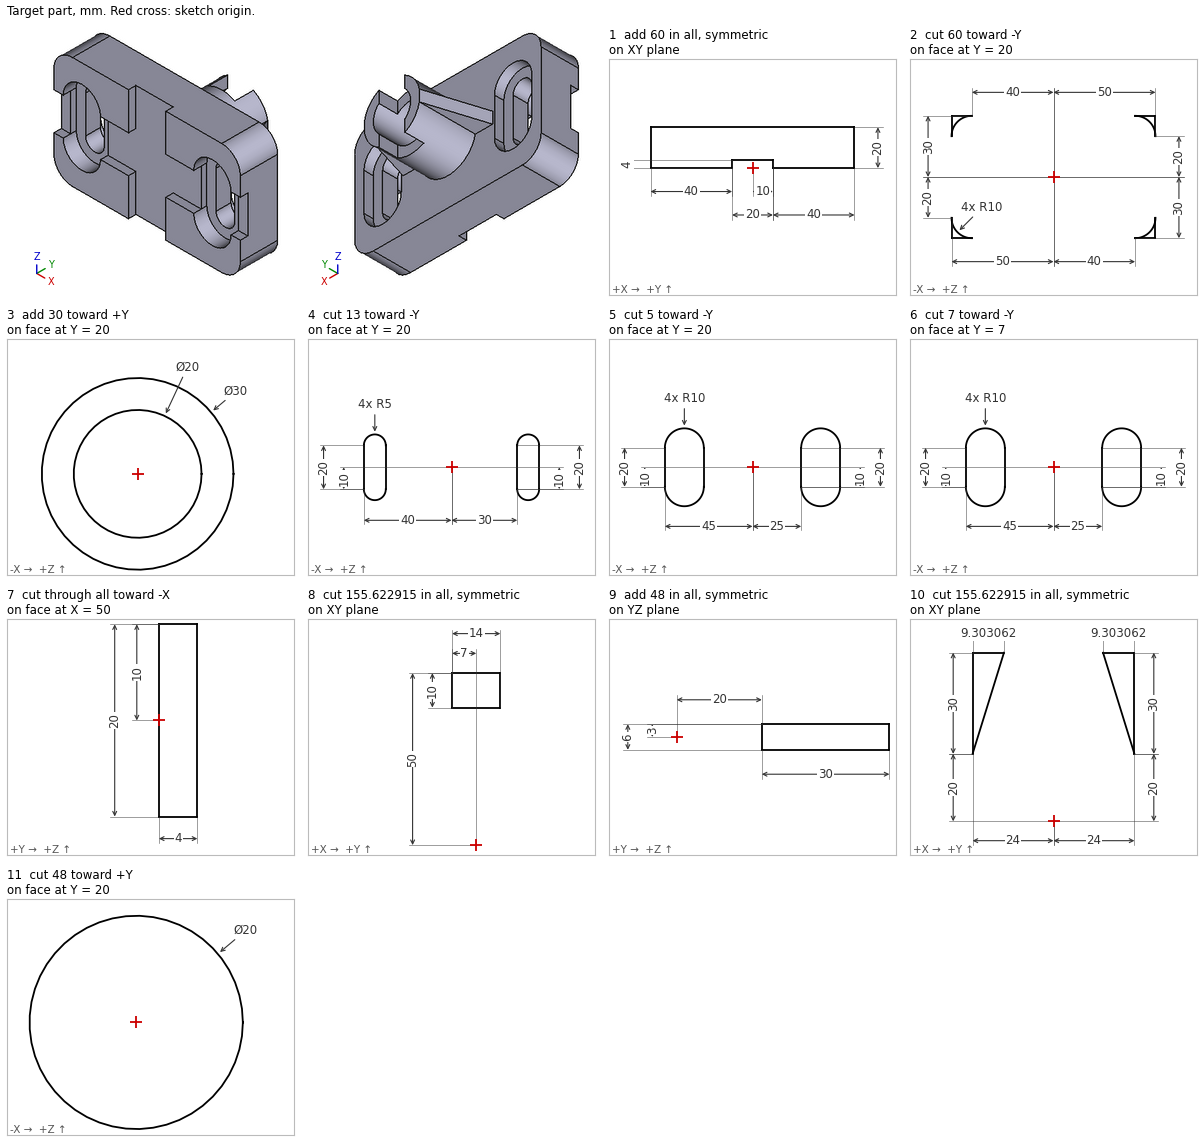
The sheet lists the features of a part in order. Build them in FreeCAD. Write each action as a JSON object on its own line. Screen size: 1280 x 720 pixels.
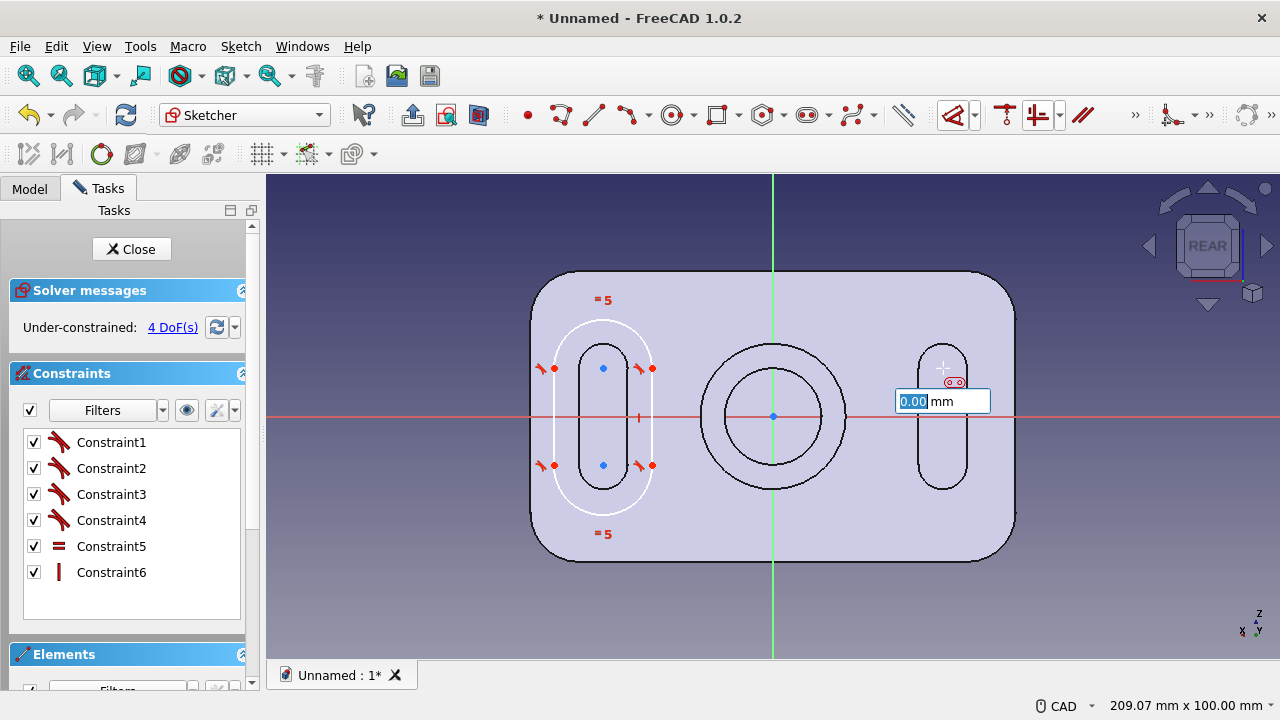
{"action": "left_click", "coordinate": [894, 402]}
{"action": "key", "text": "Escape"}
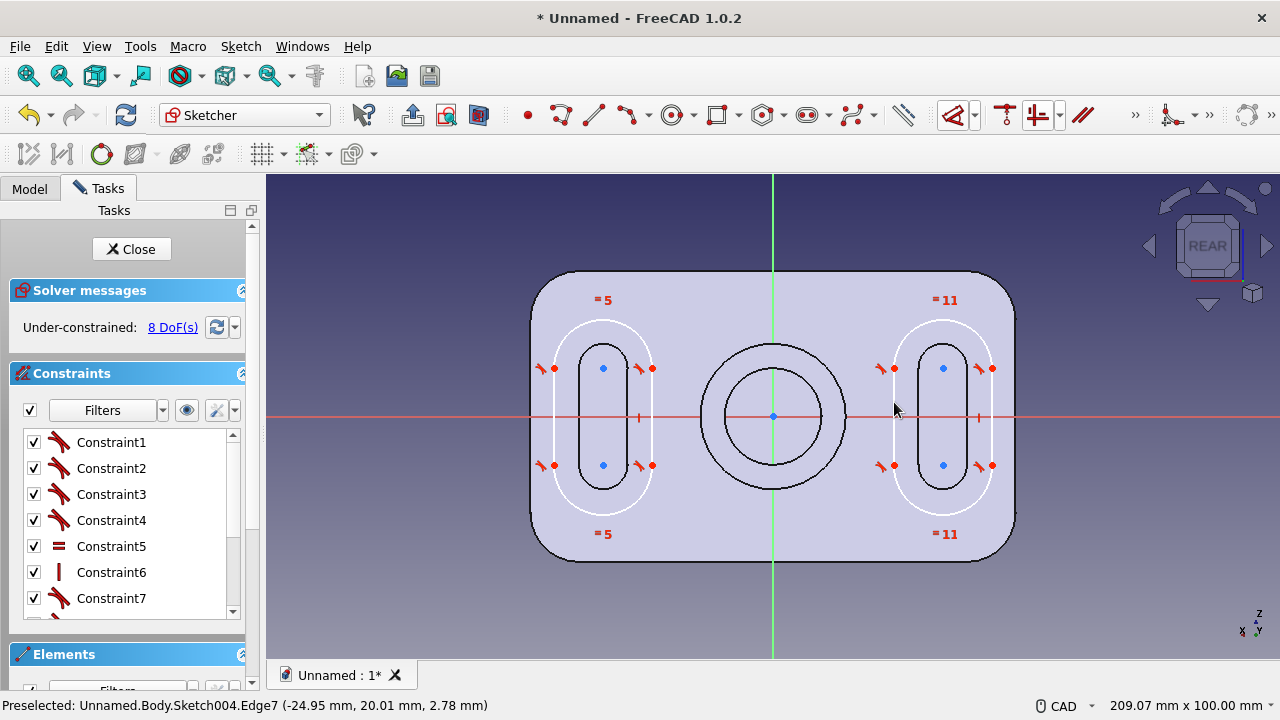
{"action": "left_click", "coordinate": [574, 506]}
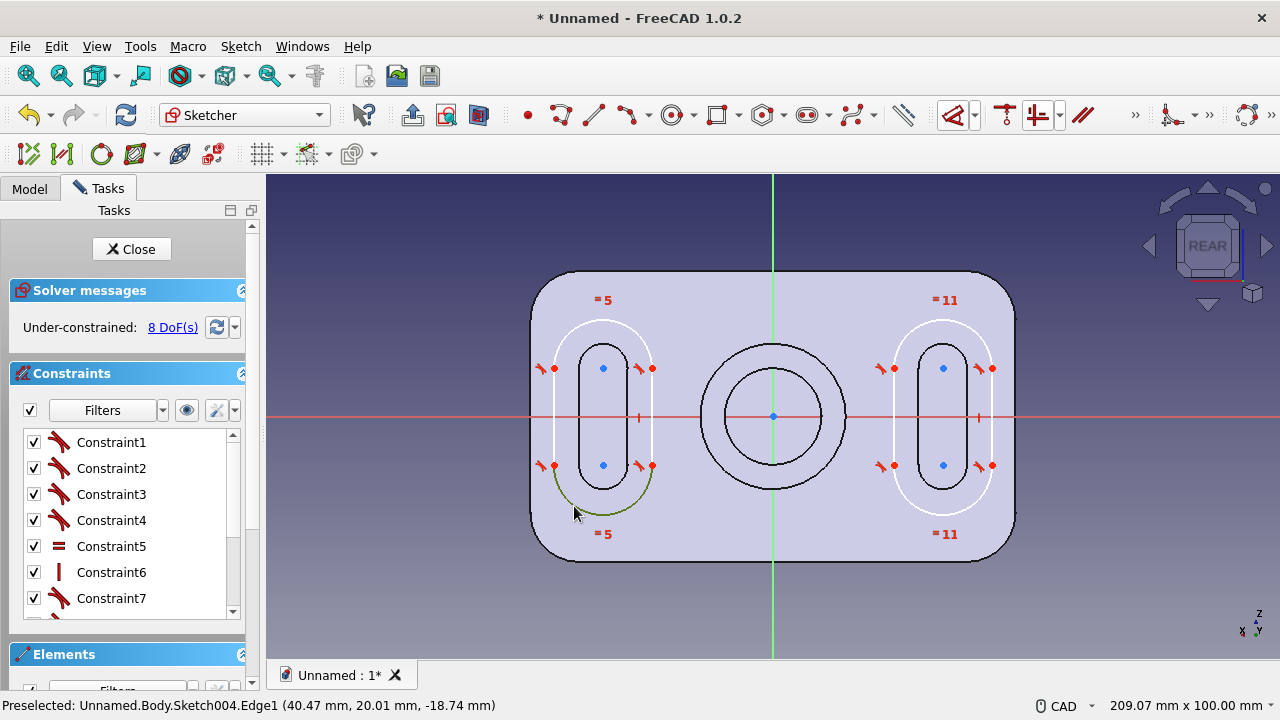
{"action": "left_click", "coordinate": [914, 506]}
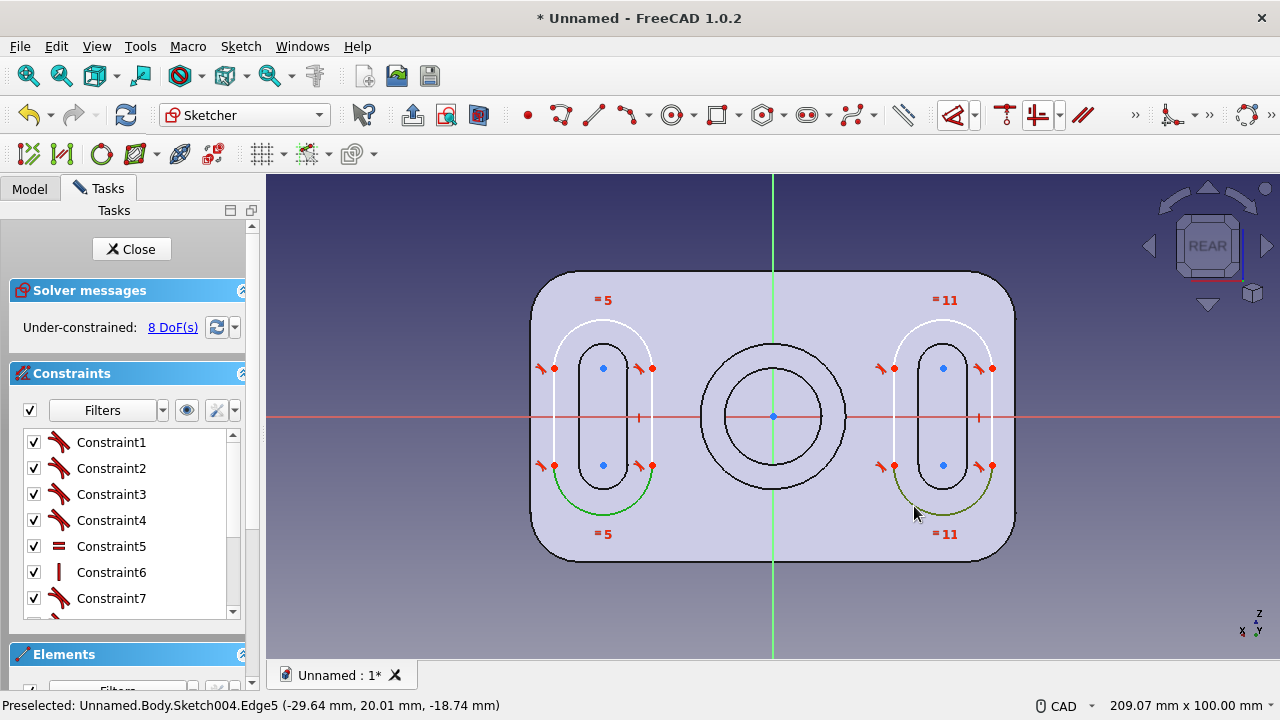
{"action": "key", "text": "e"}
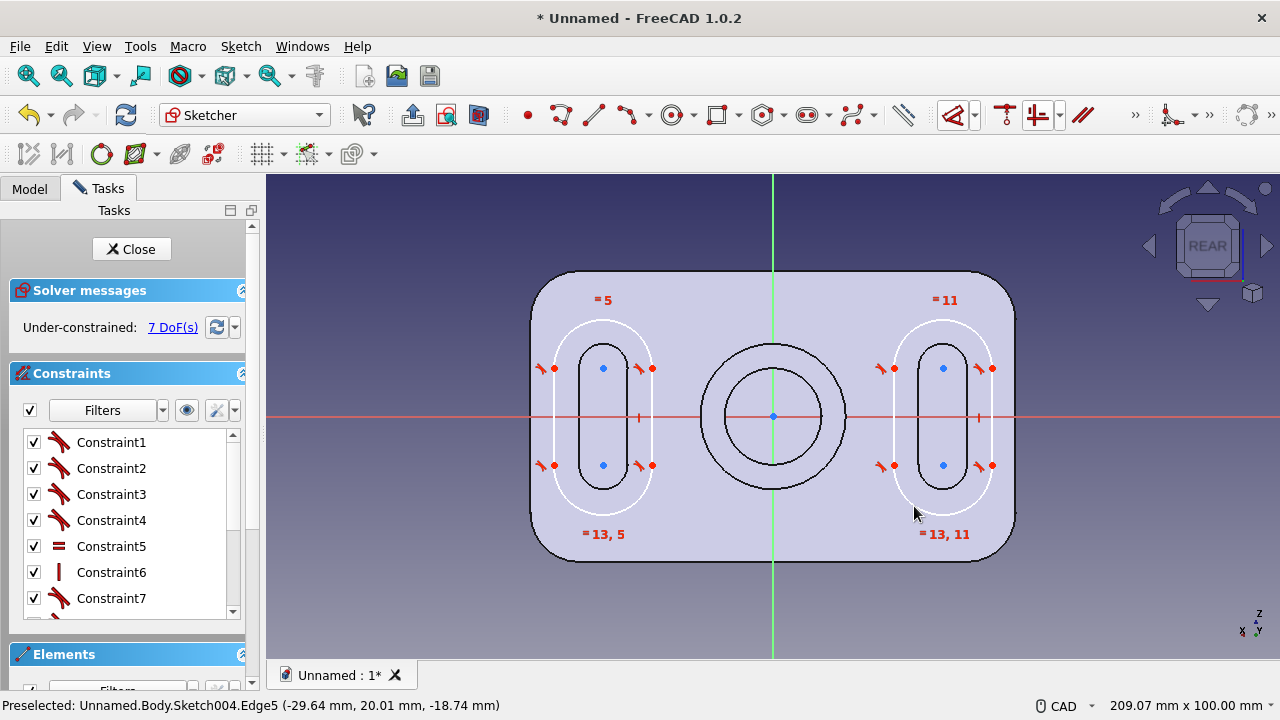
{"action": "left_click", "coordinate": [574, 506]}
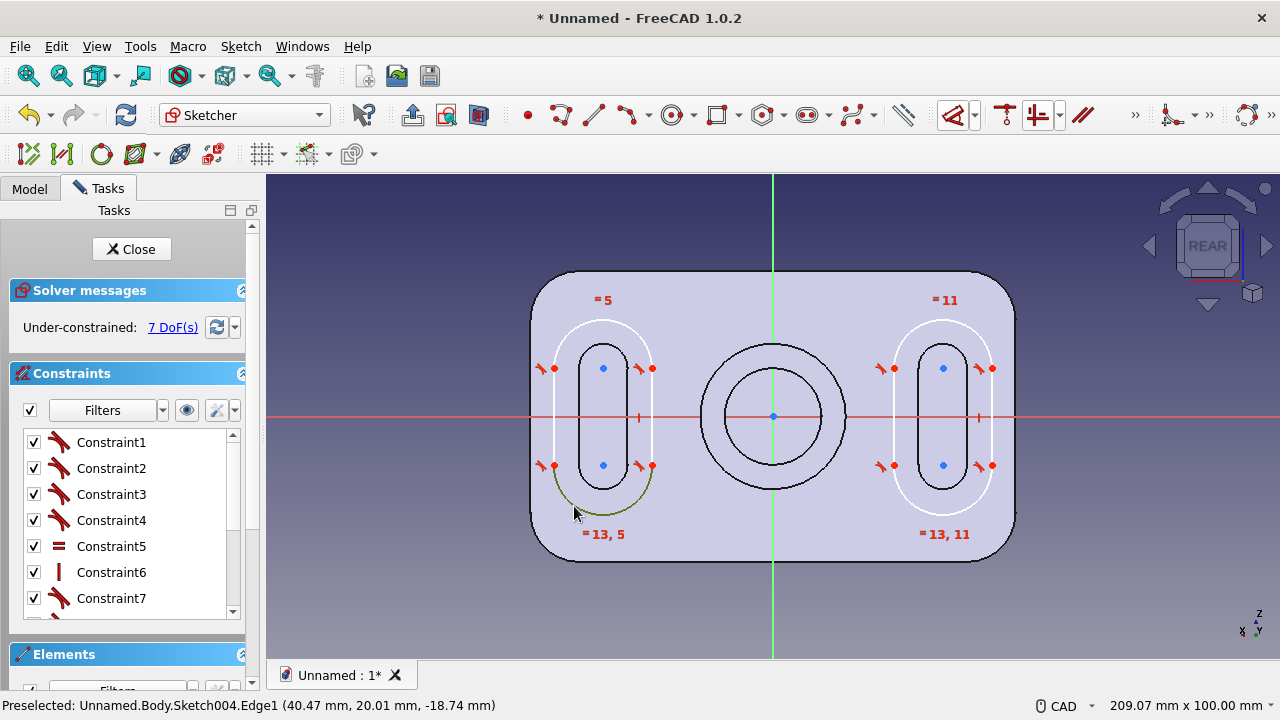
{"action": "key", "text": "k r"}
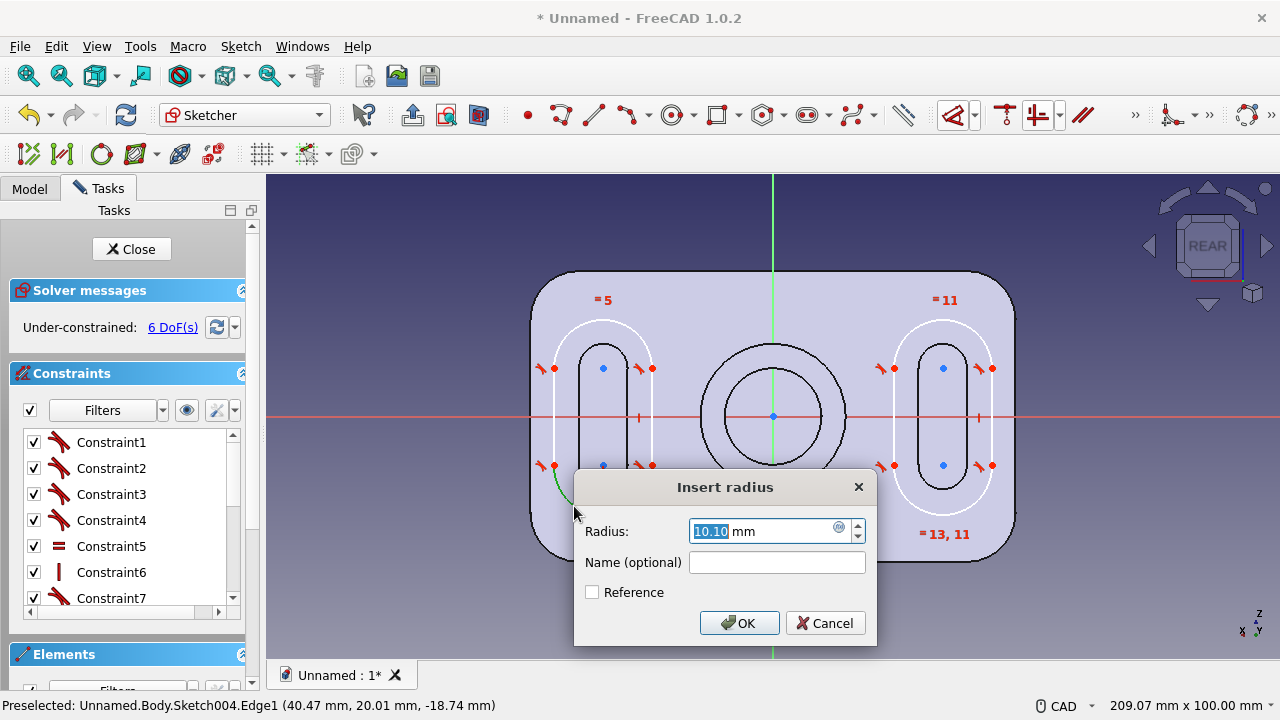
{"action": "type", "text": "10"}
{"action": "key", "text": "Return"}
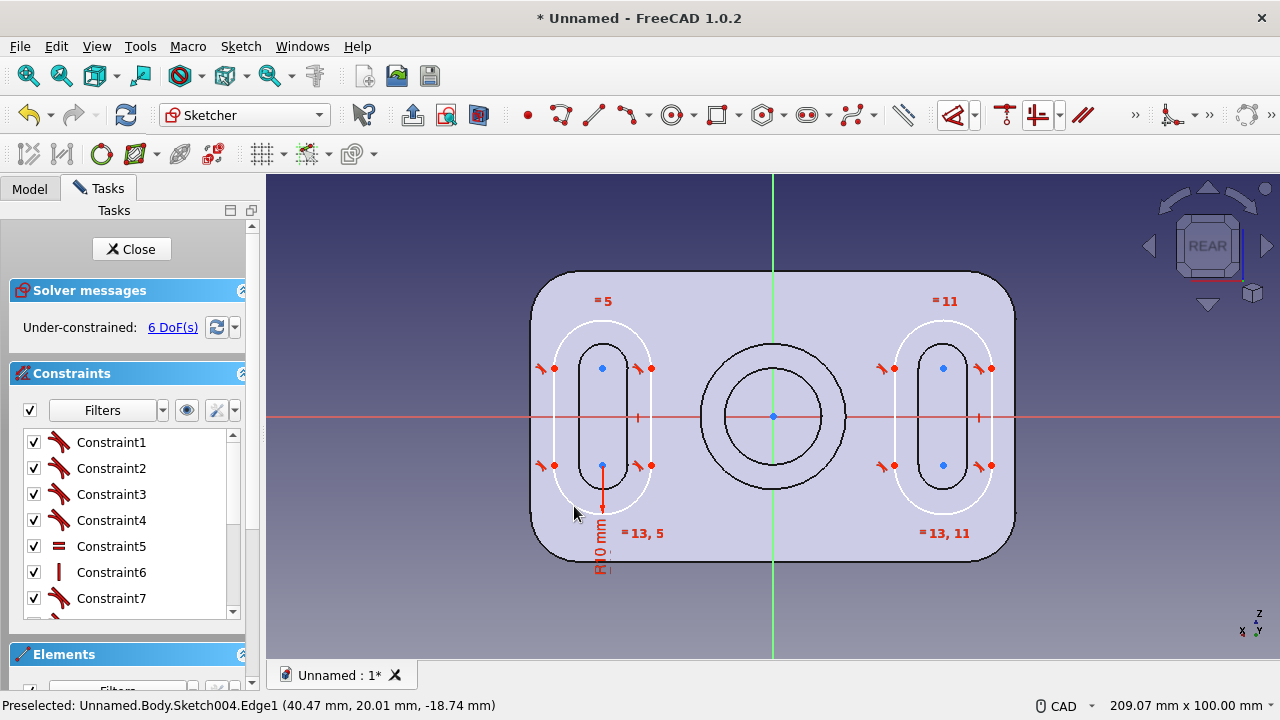
{"action": "left_click", "coordinate": [554, 437]}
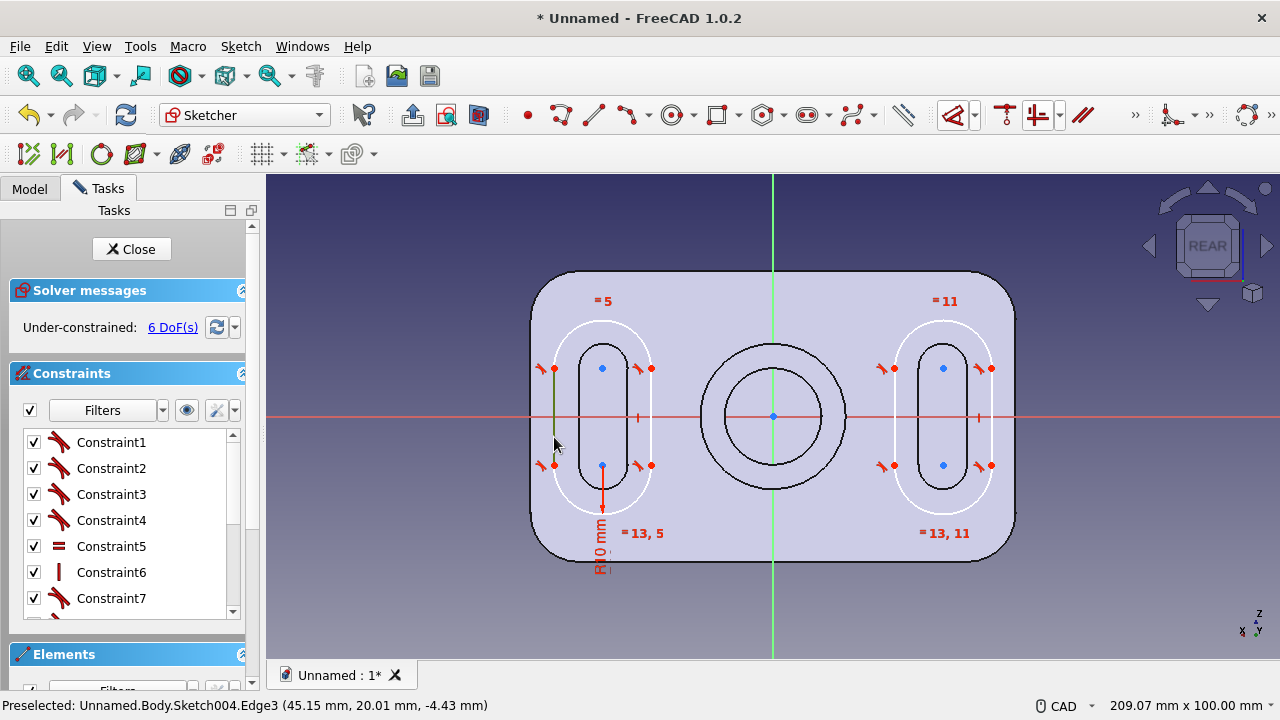
{"action": "key", "text": "i"}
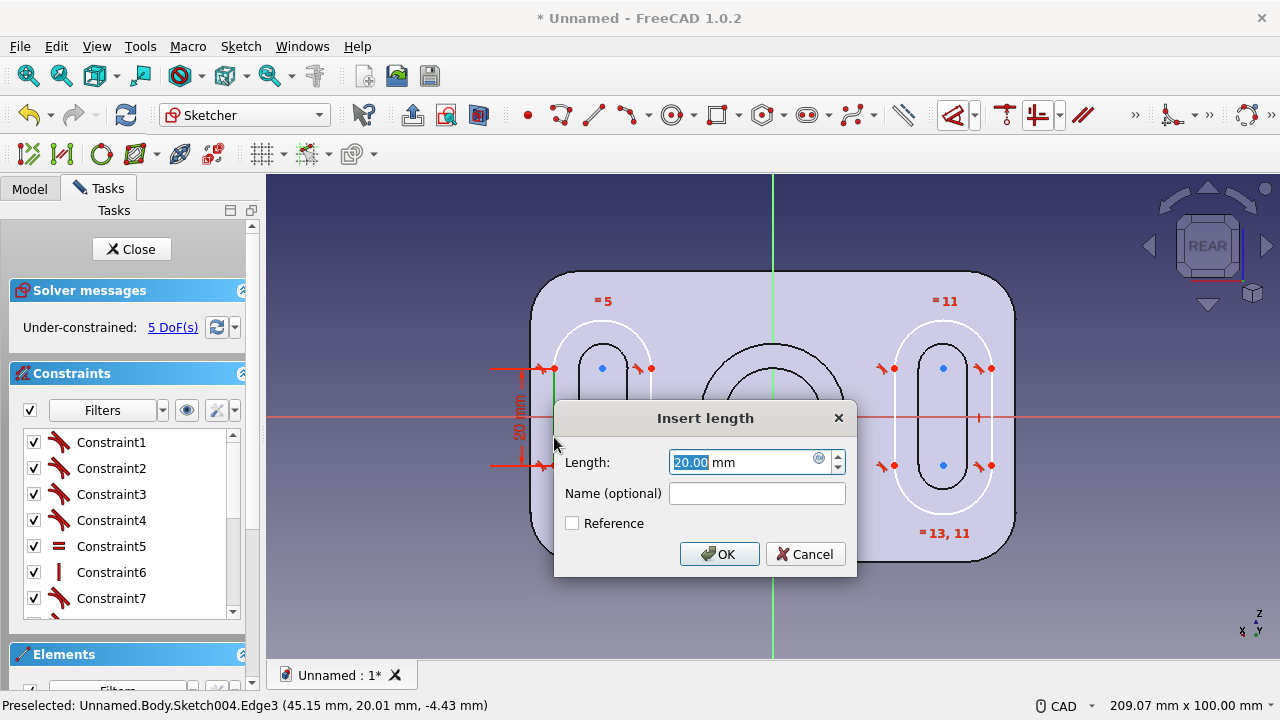
{"action": "type", "text": "20"}
{"action": "key", "text": "Return"}